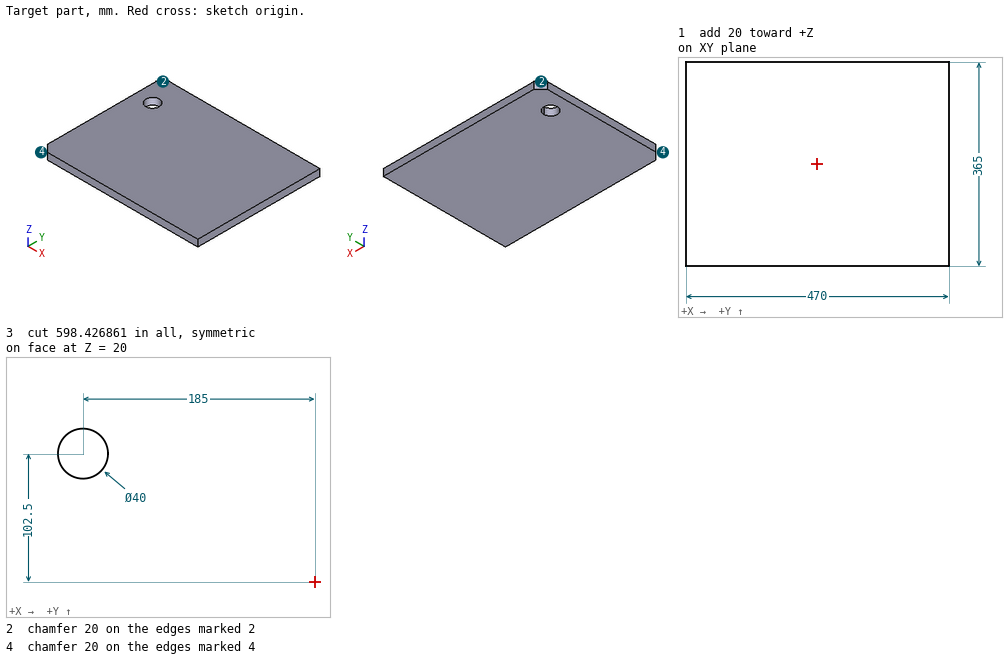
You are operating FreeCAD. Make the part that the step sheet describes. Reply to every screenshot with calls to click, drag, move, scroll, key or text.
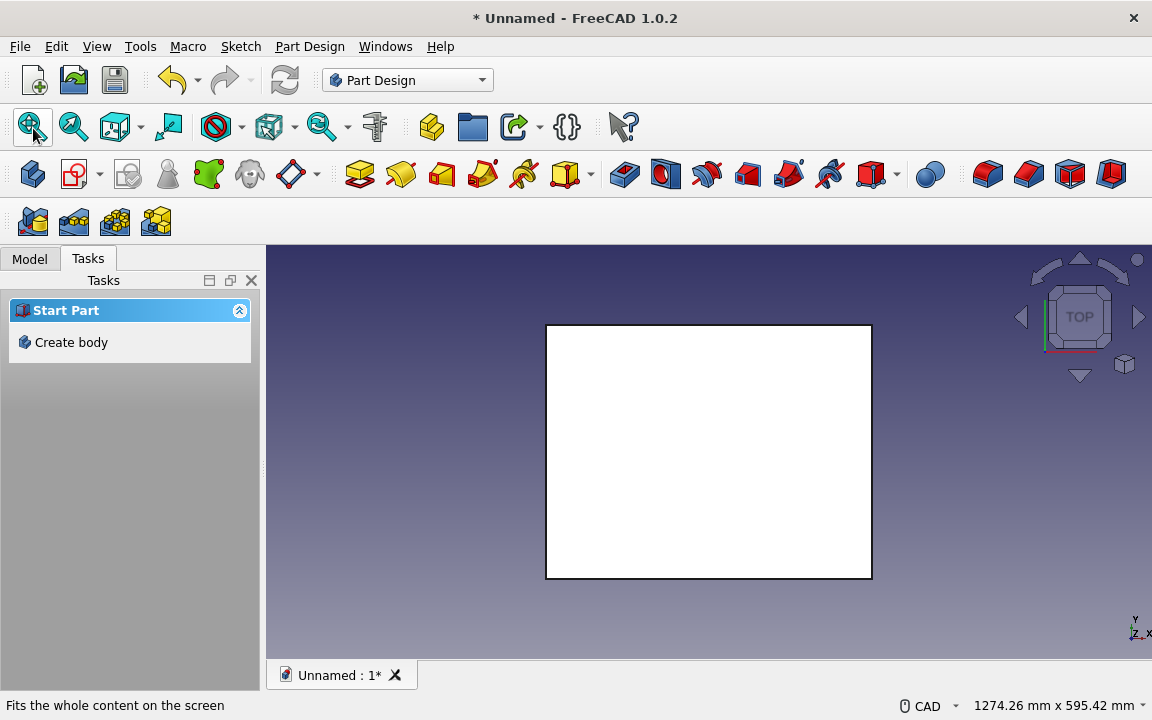
scroll(546, 324, up, 6)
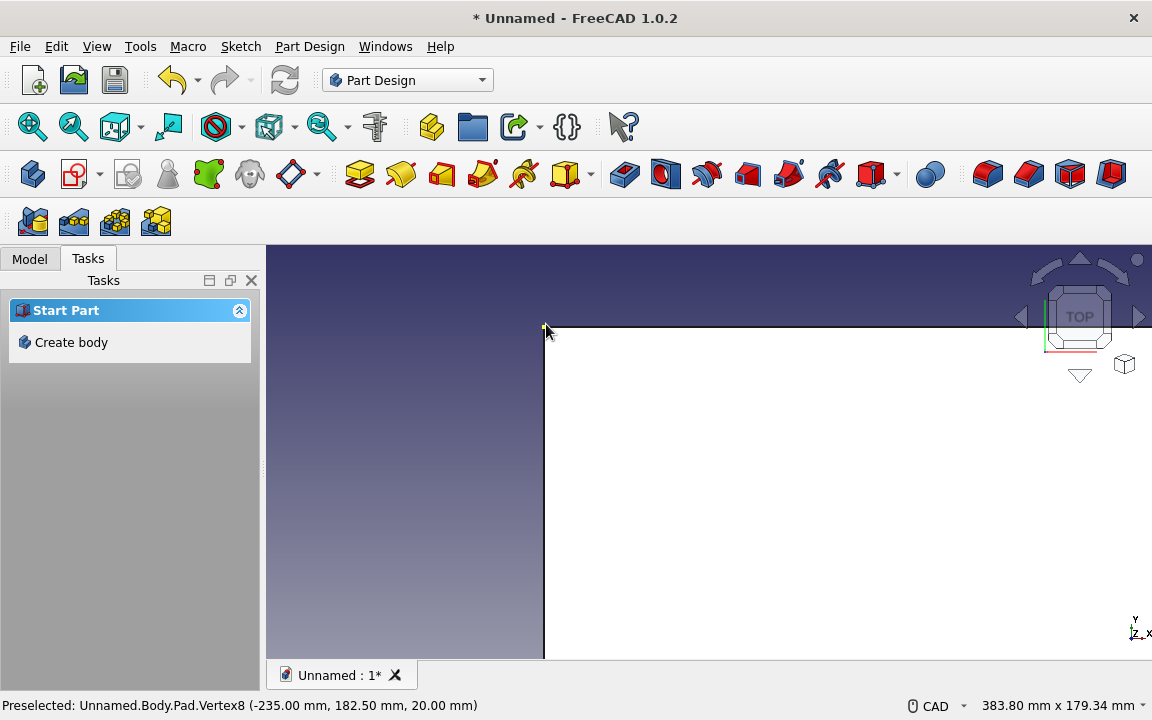
click(33, 128)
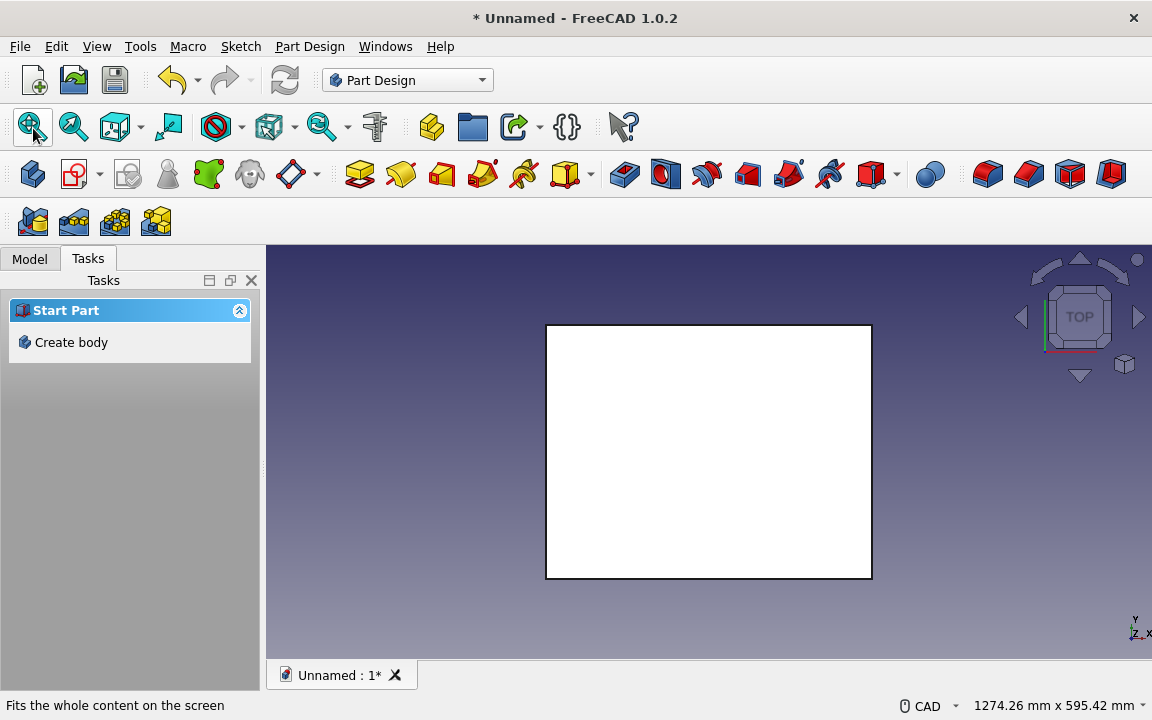
key(1)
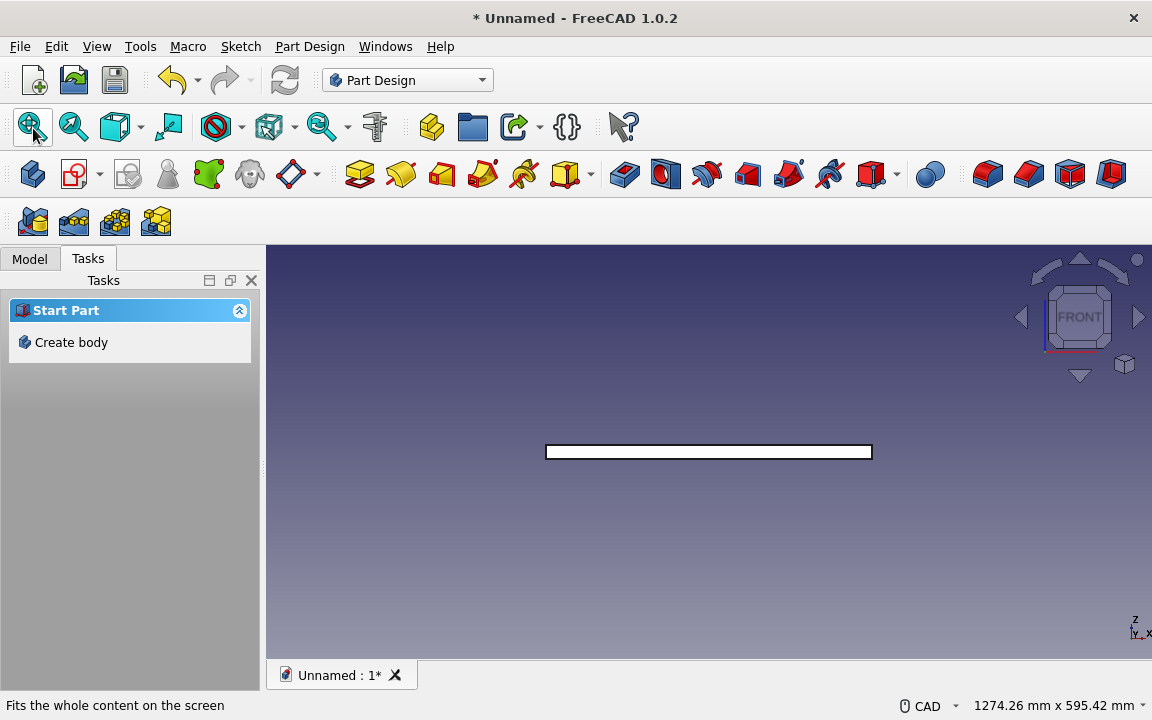
click(33, 128)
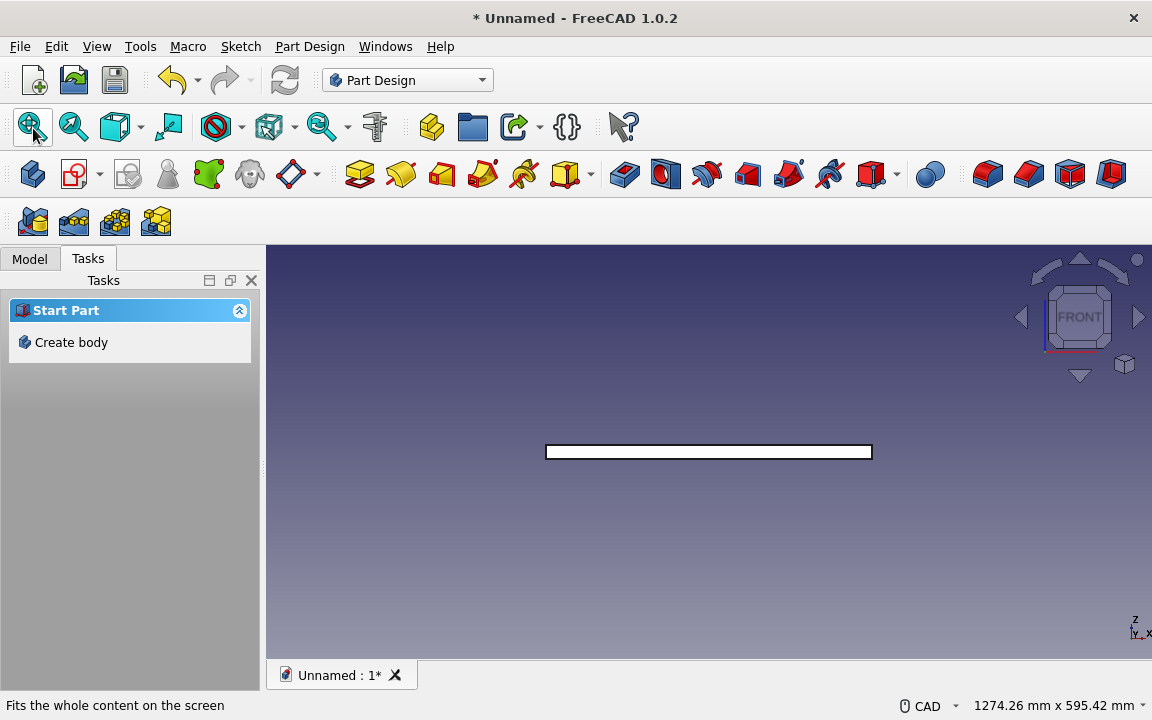
scroll(546, 451, up, 6)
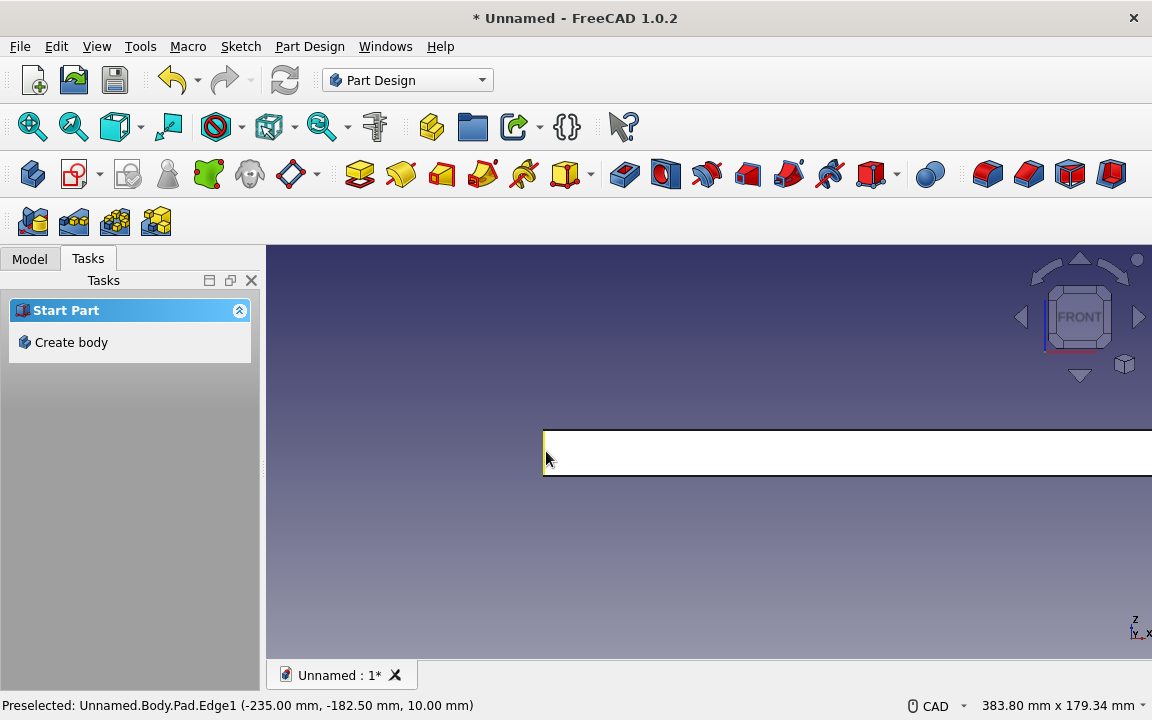
click(33, 128)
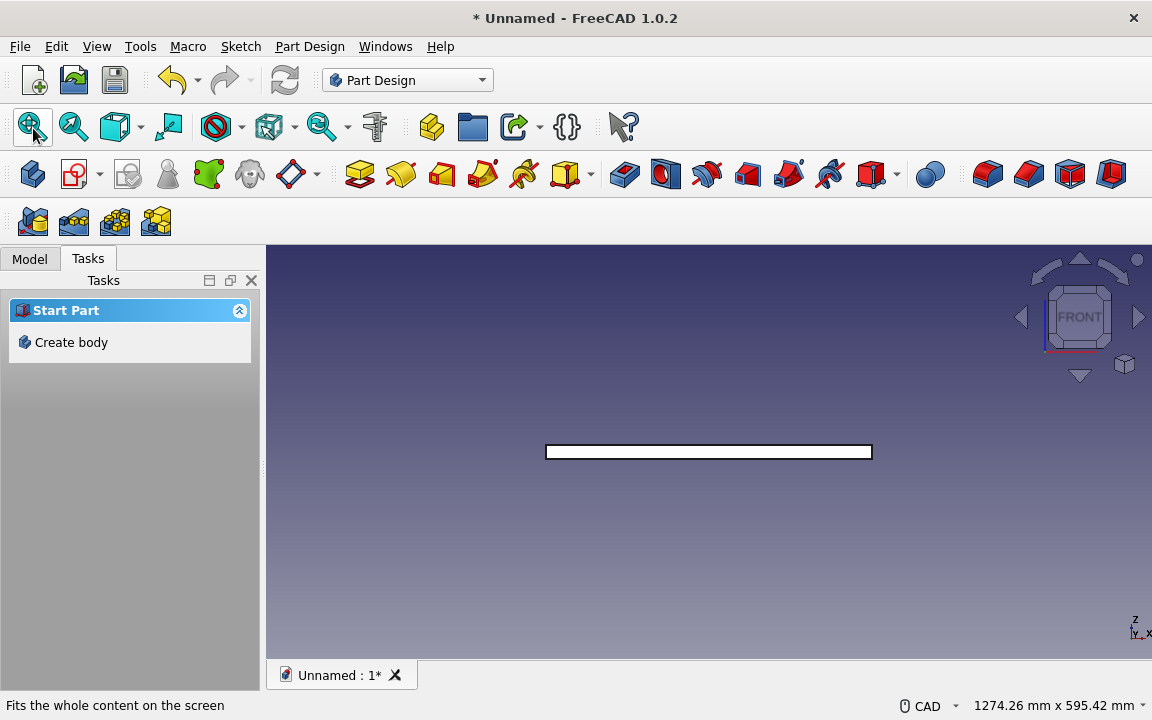
key(3)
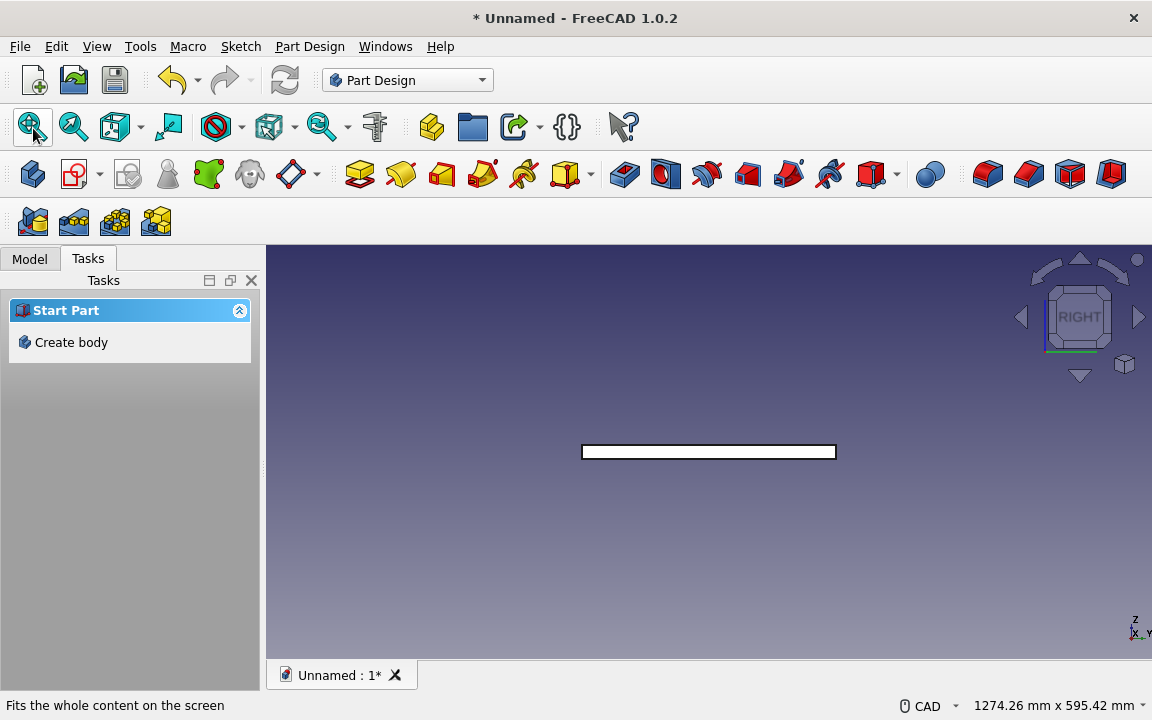
click(33, 128)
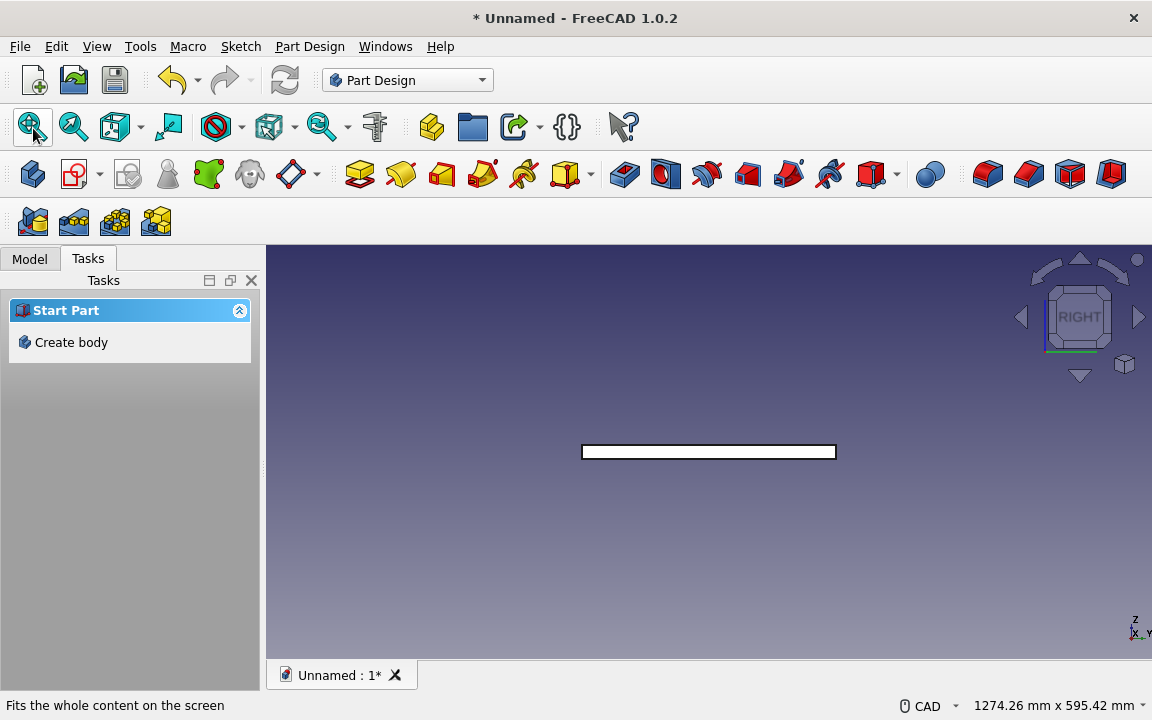
scroll(836, 451, up, 6)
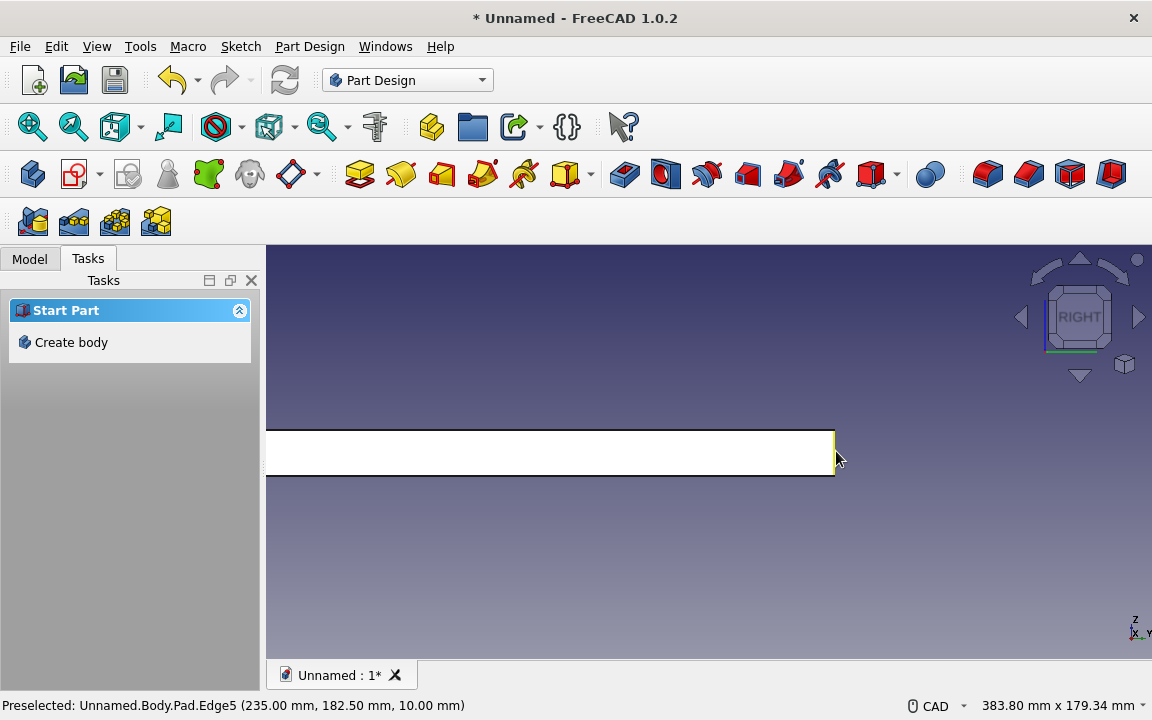
click(33, 128)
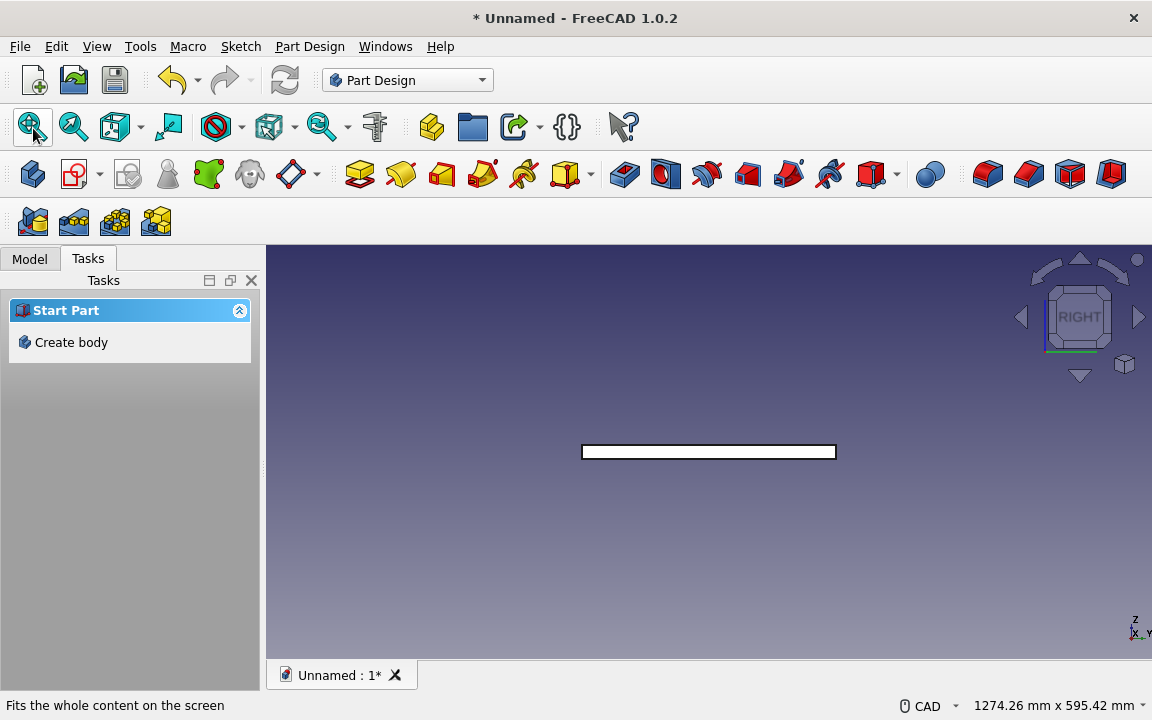
key(5)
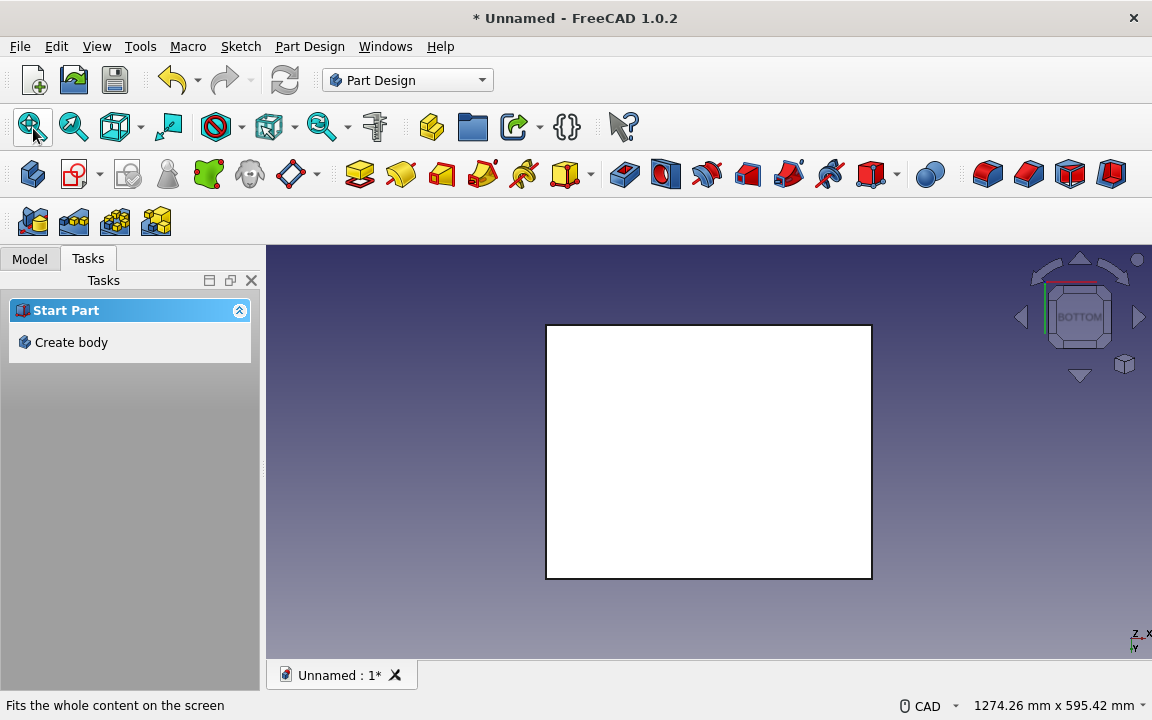
scroll(546, 578, up, 6)